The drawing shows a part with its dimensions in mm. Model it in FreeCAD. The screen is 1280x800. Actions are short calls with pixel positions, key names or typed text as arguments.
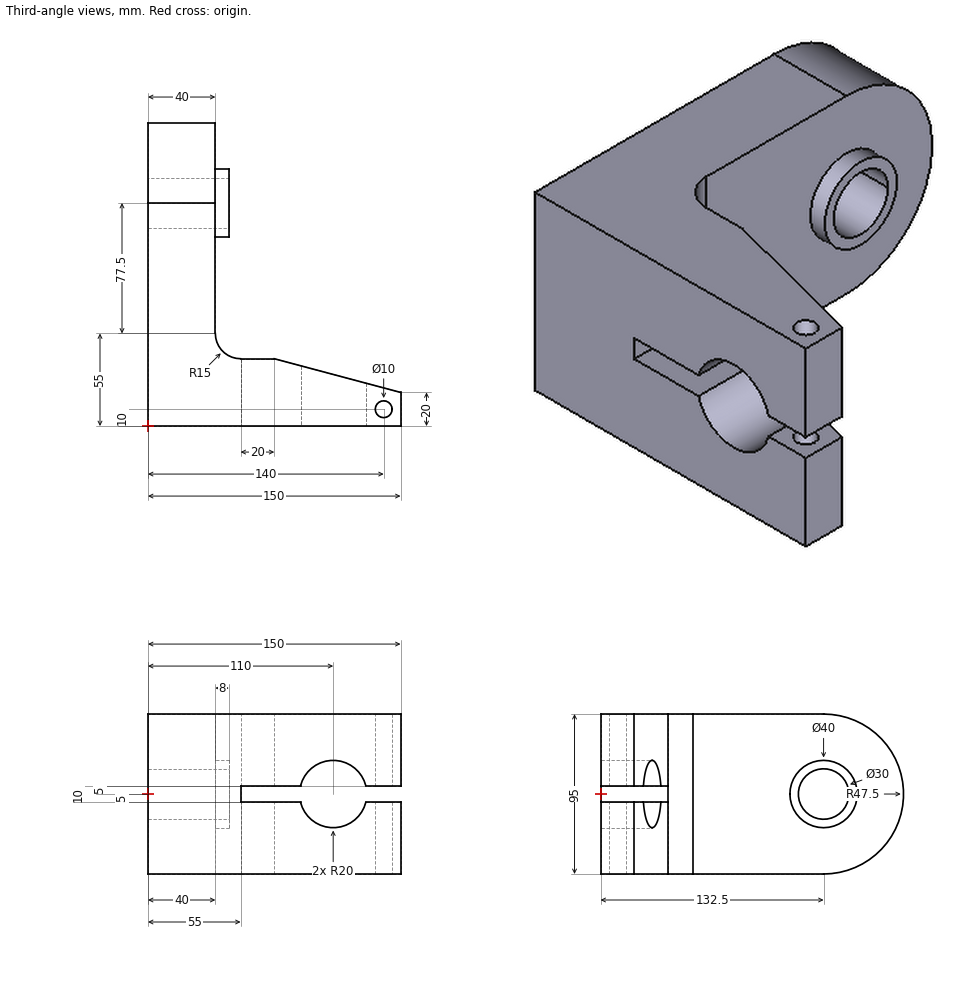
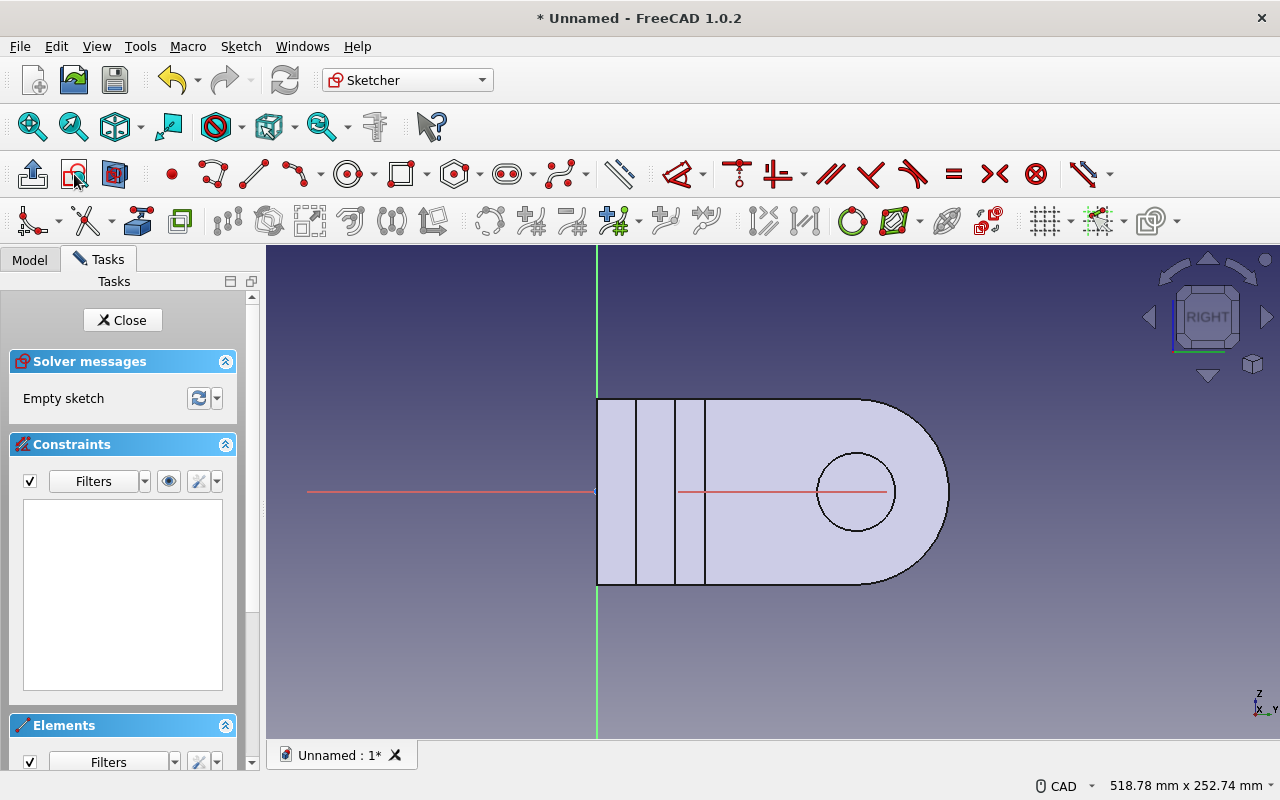
click(115, 174)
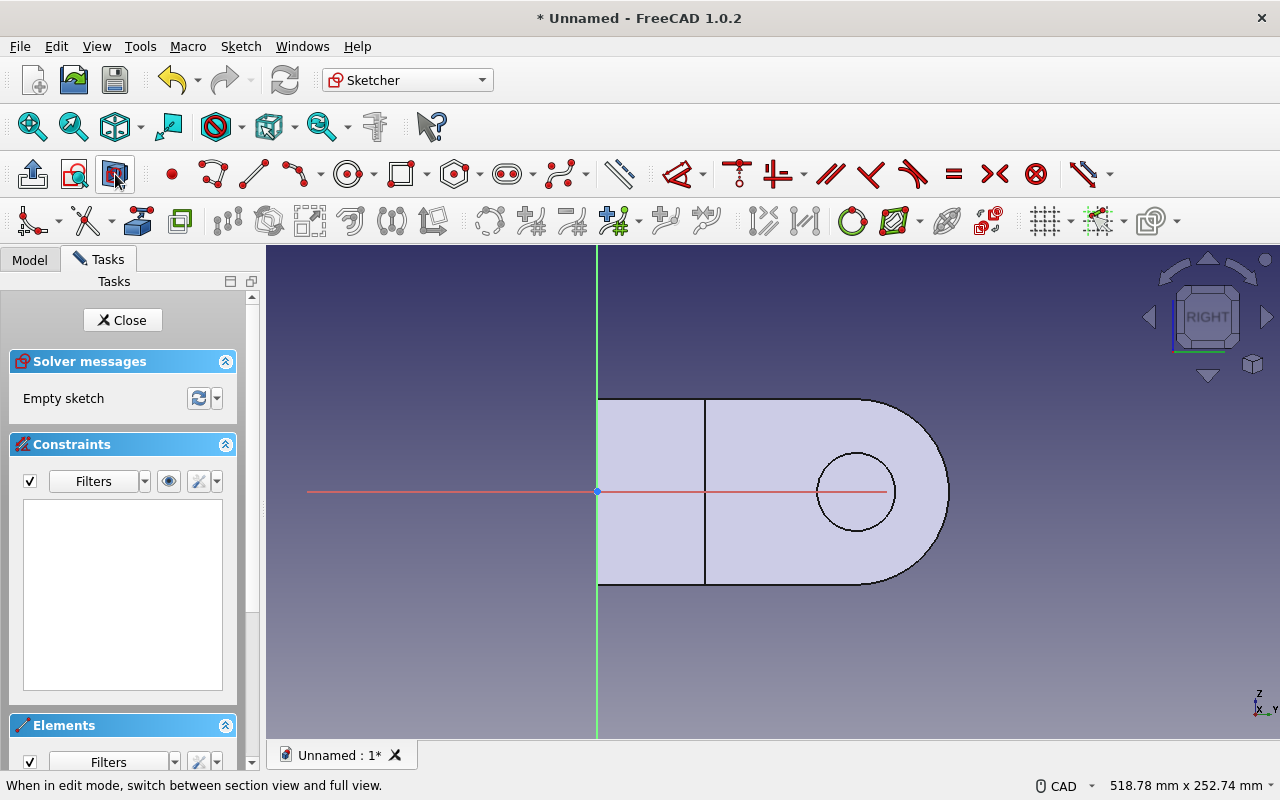
scroll(895, 492, up, 8)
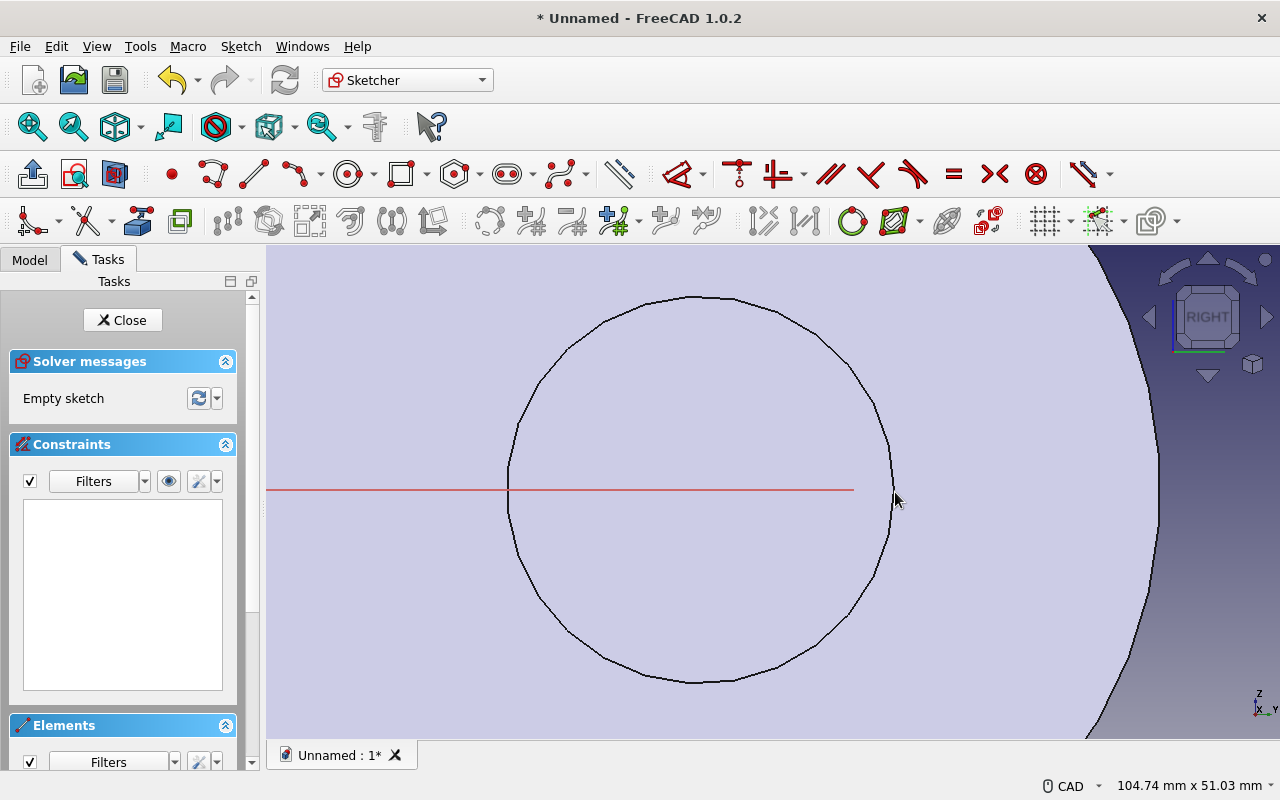
click(348, 174)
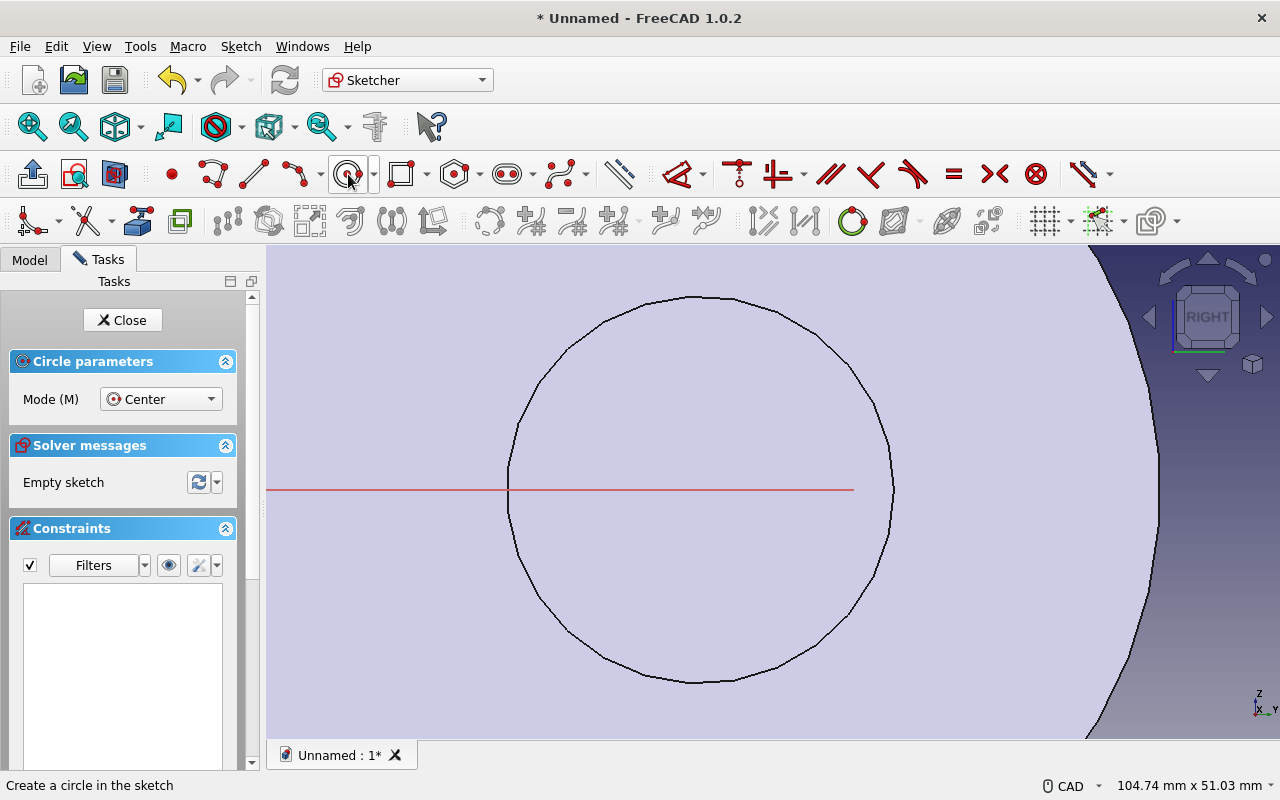
click(700, 490)
move(803, 387)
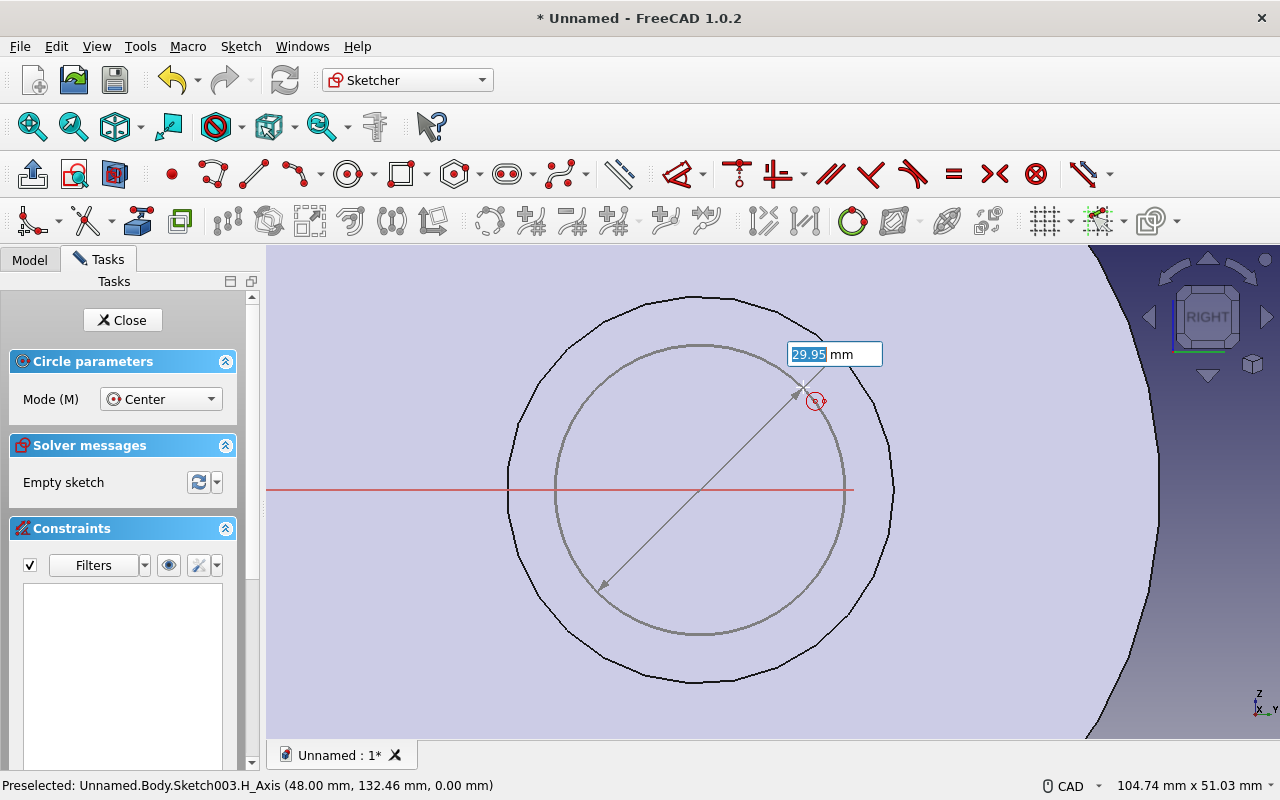
text(30)
key(Return)
key(Escape)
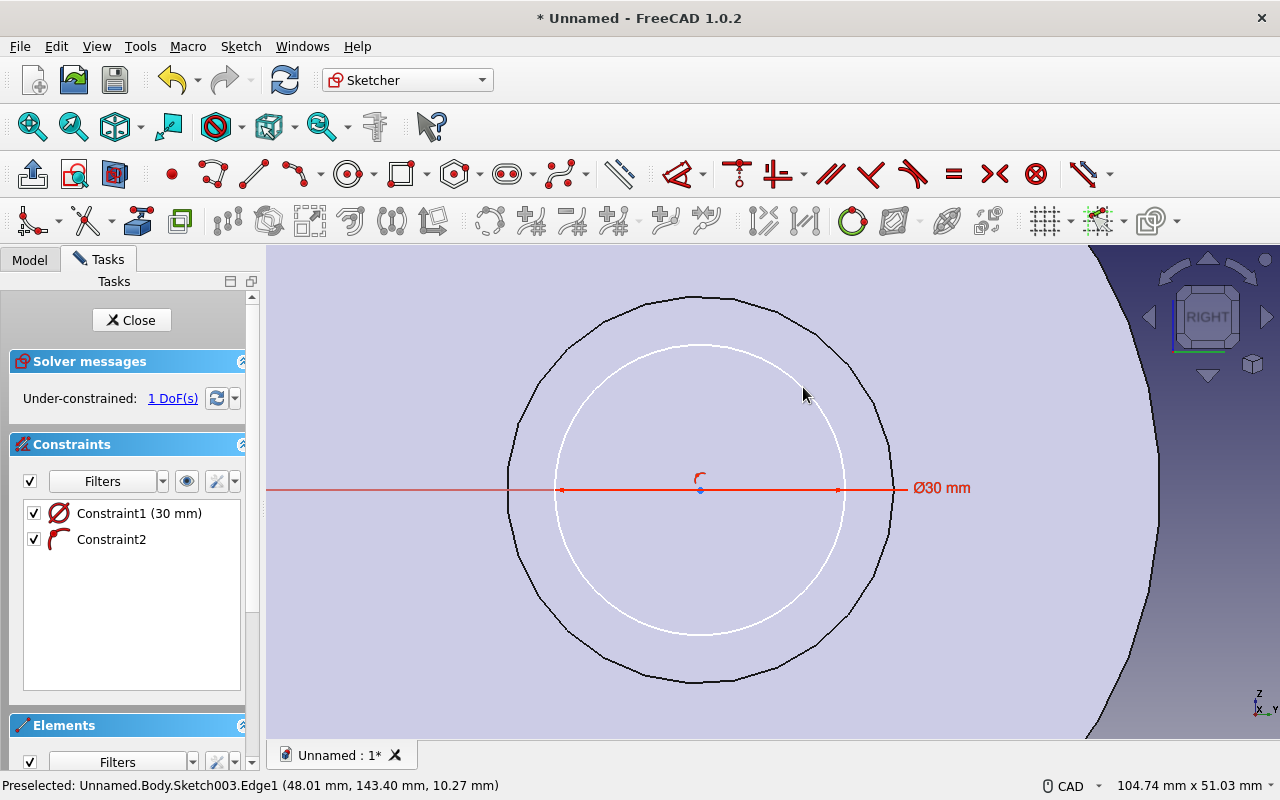
click(676, 174)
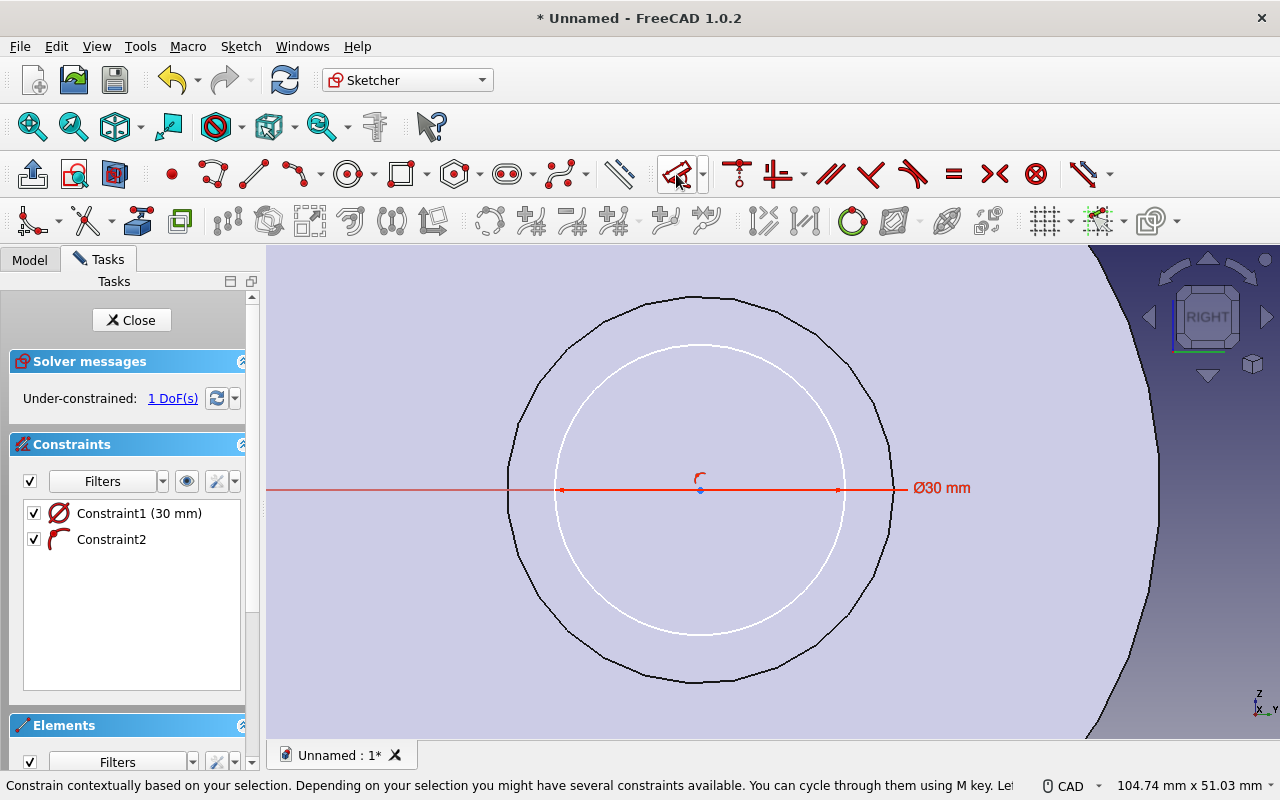
click(700, 490)
click(497, 524)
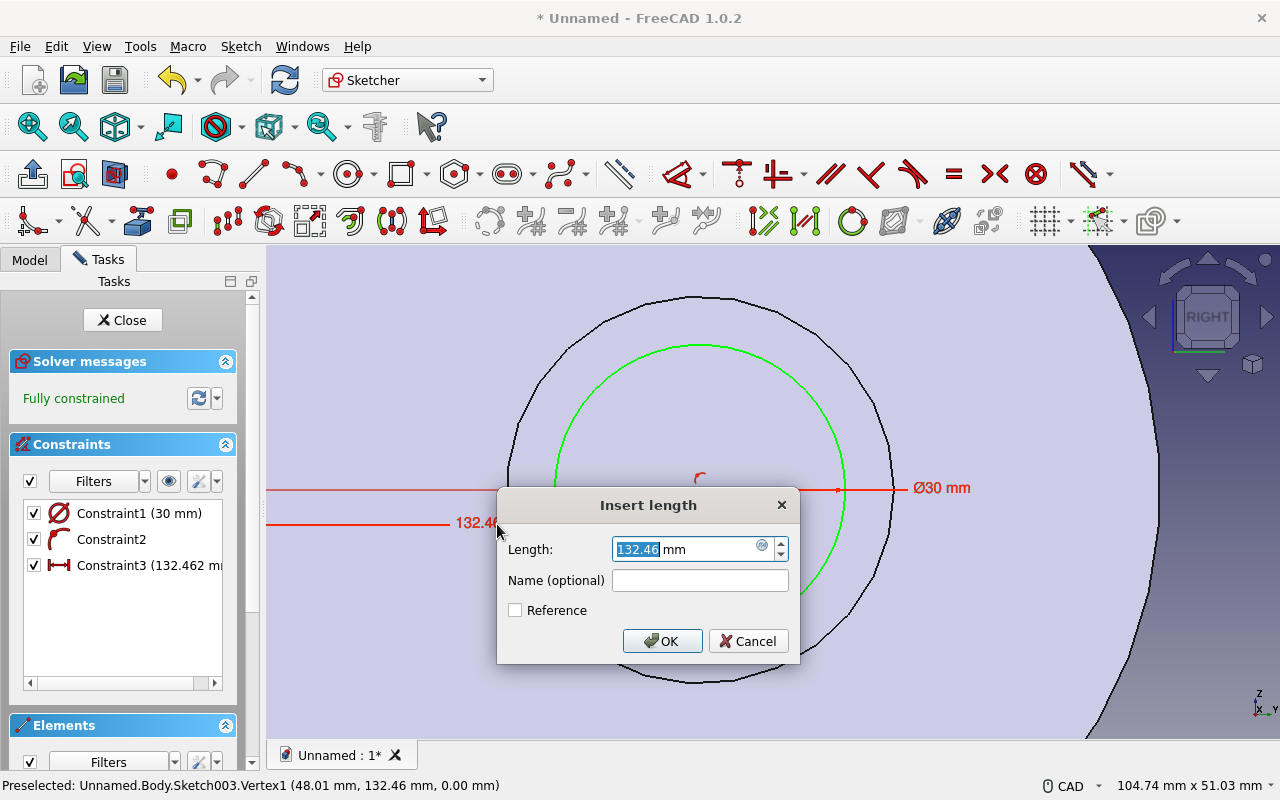
text(132.5)
key(Return)
key(Escape)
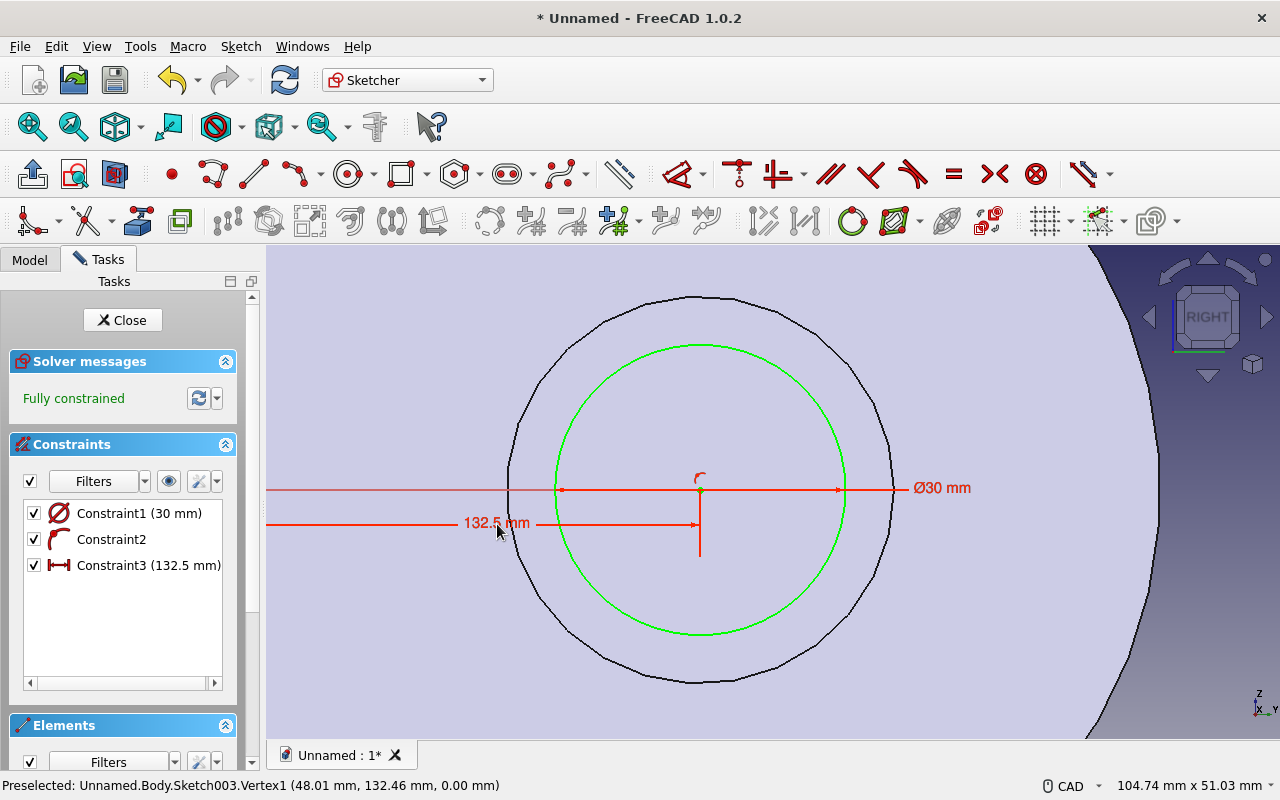
click(123, 320)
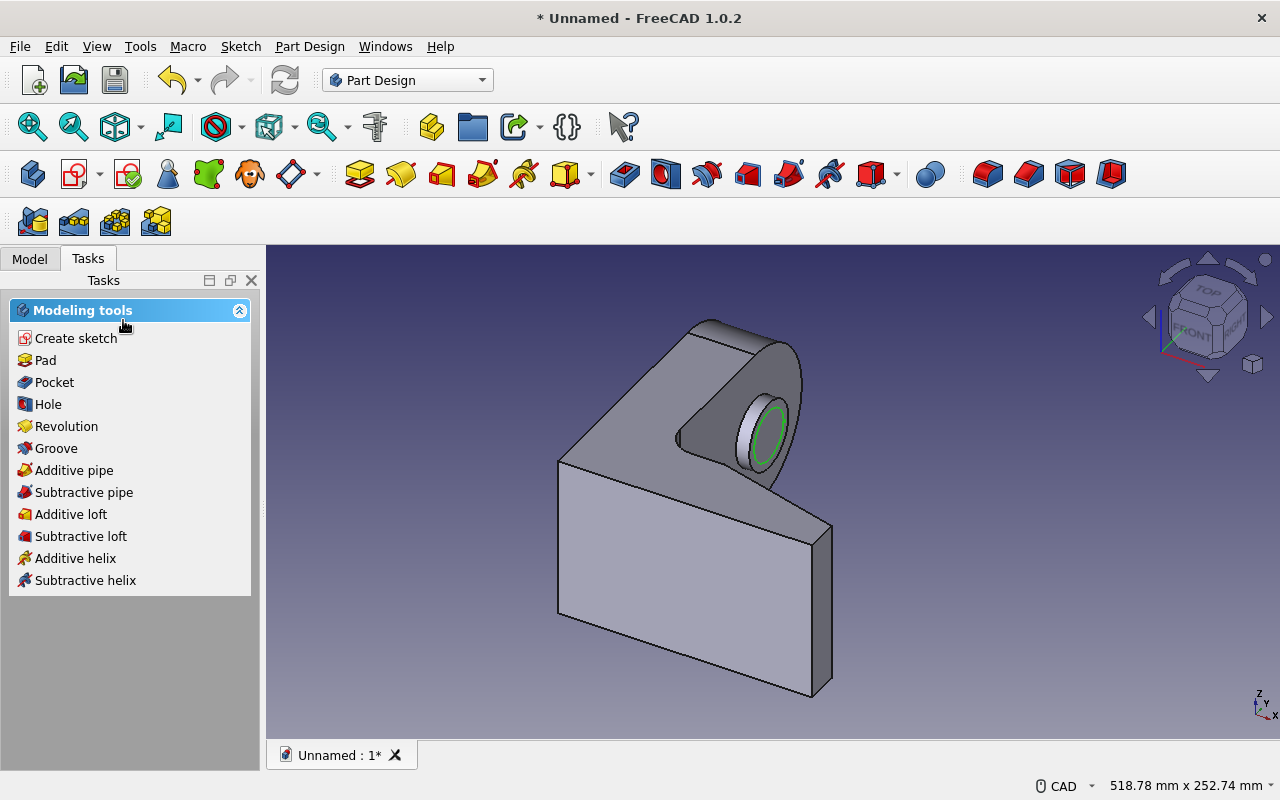
click(625, 174)